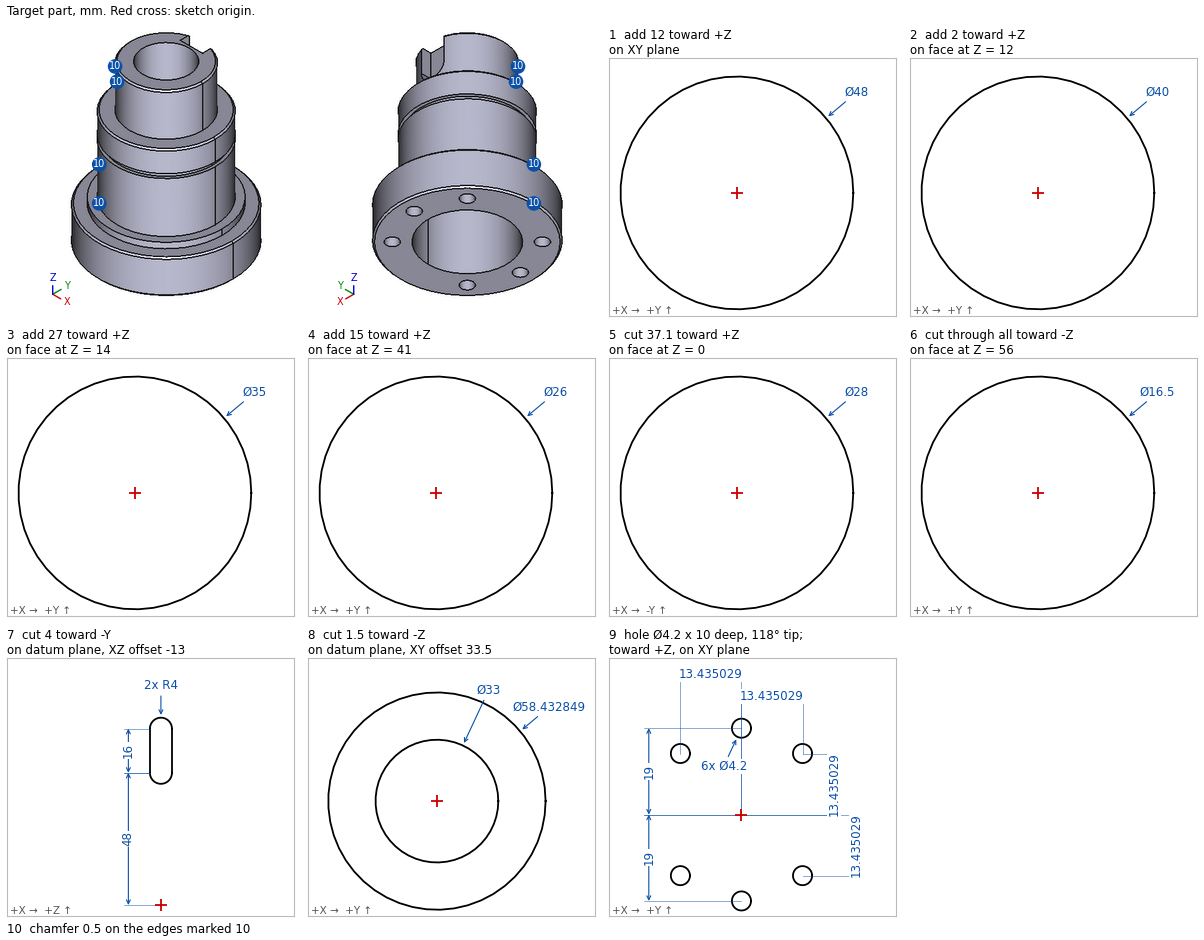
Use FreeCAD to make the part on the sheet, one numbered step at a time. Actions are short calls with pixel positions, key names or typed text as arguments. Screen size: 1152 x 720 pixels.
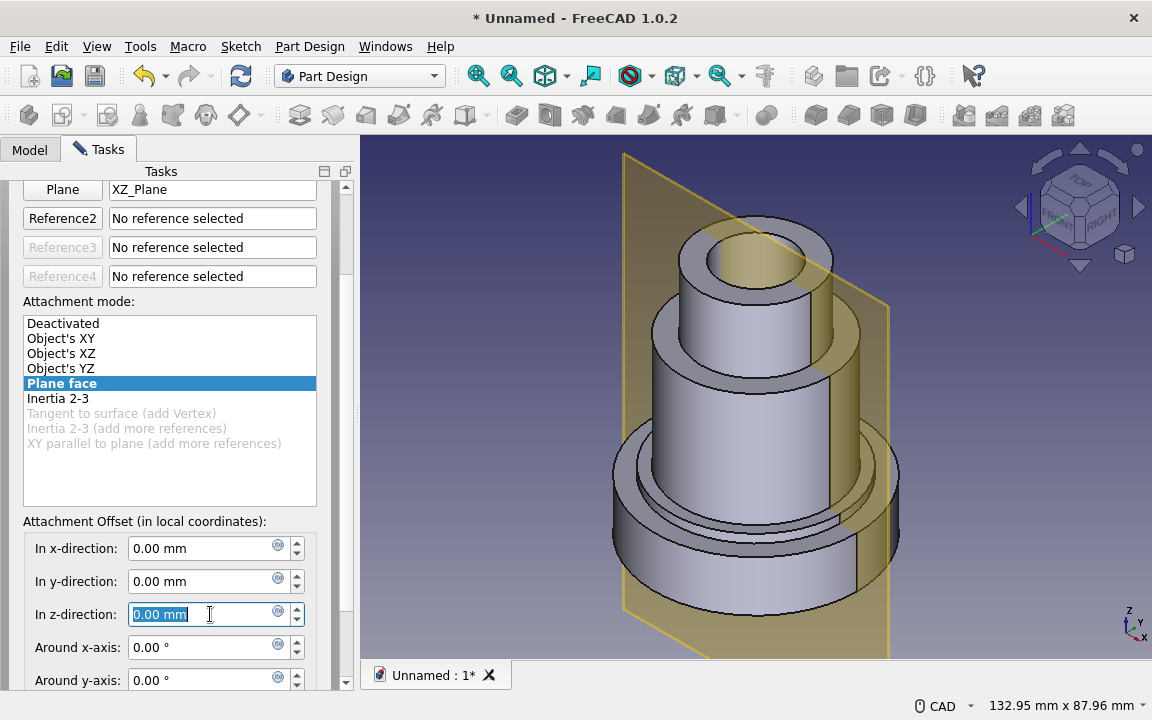
text(-13)
key(Tab)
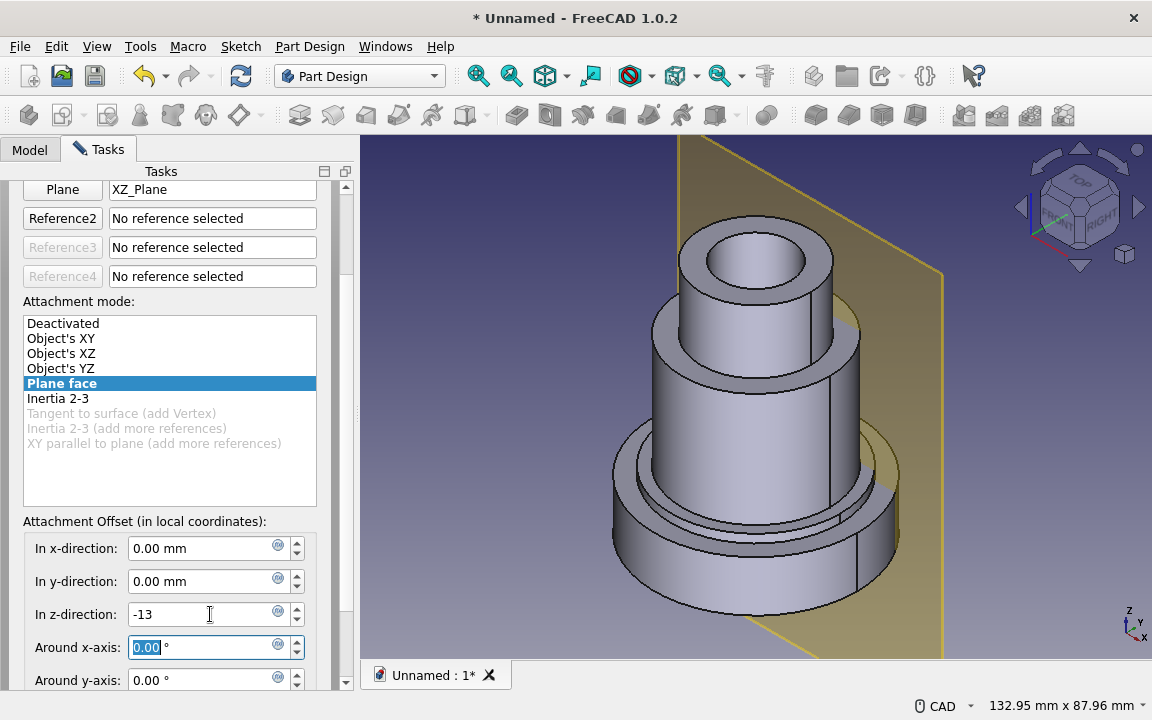
scroll(346, 436, up, 3)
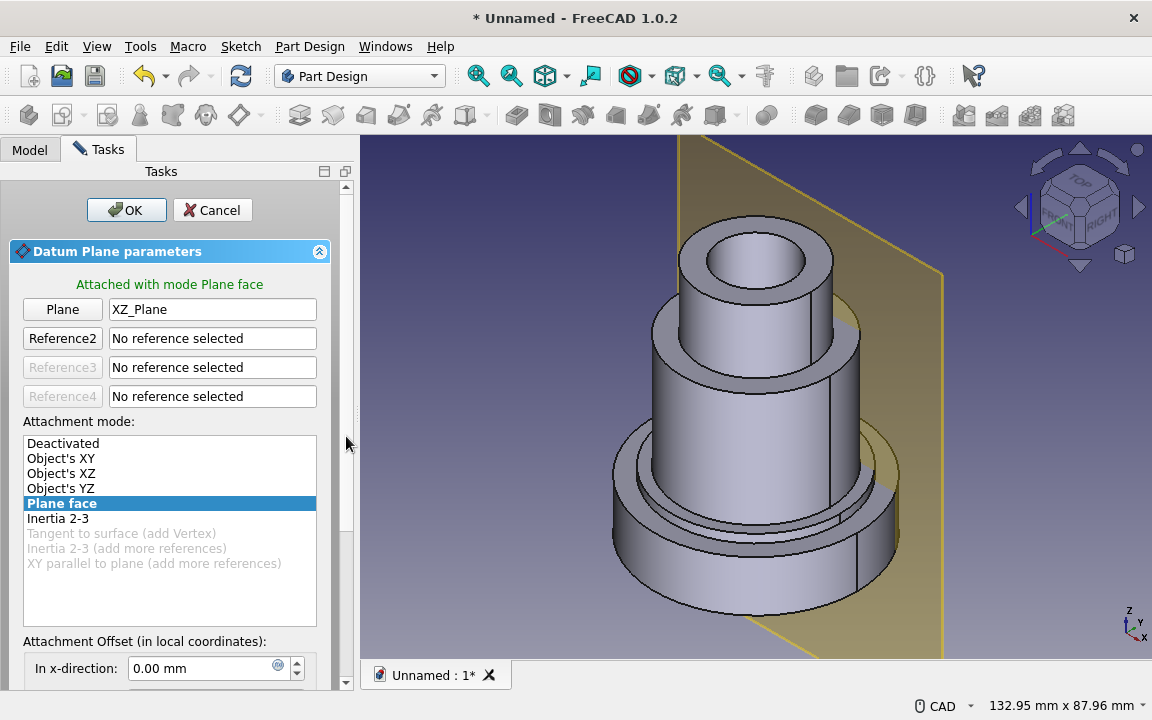
click(127, 210)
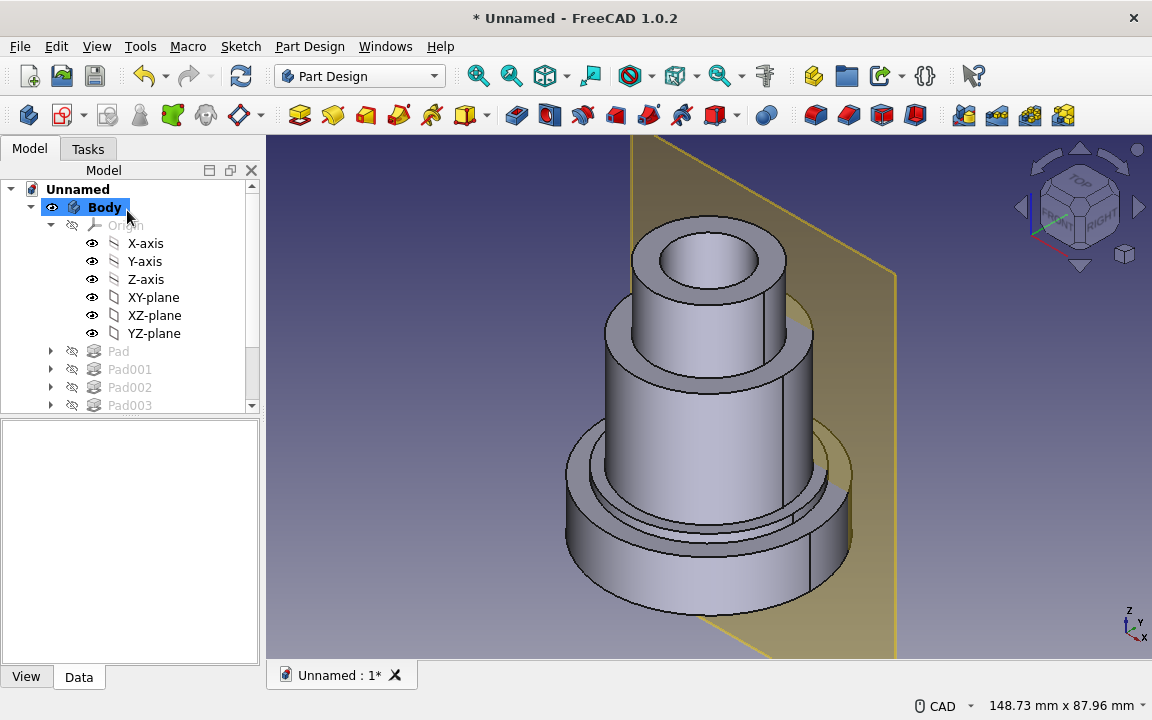
scroll(101, 293, down, 3)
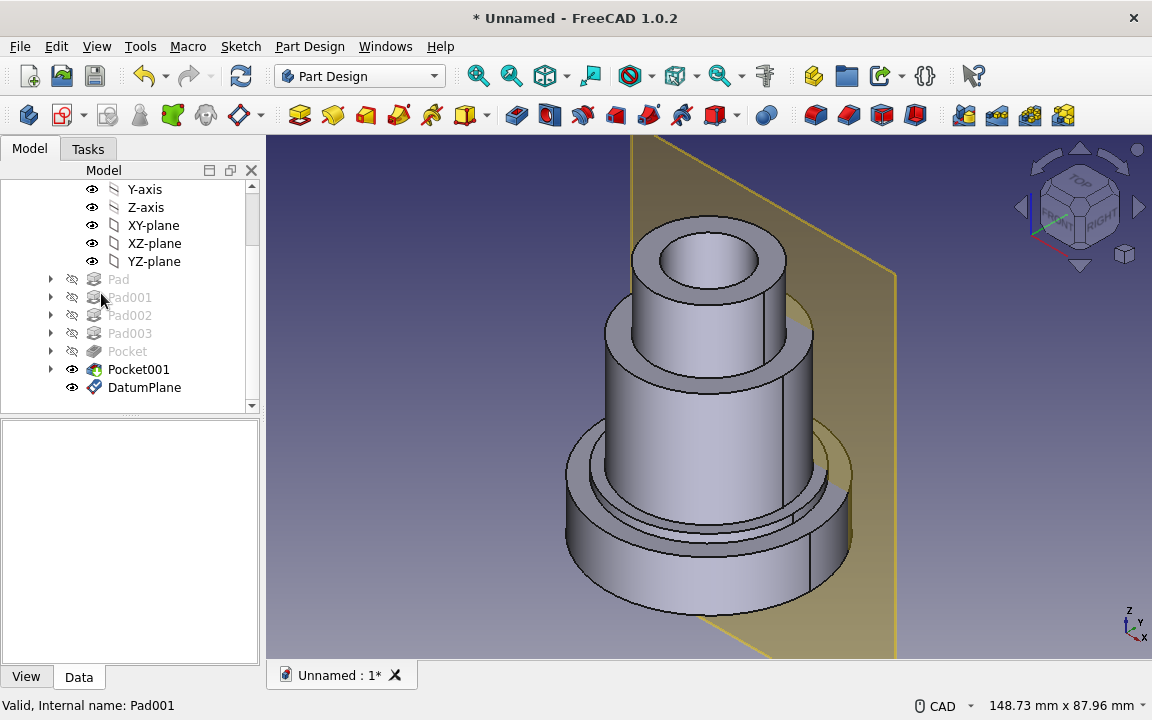
click(117, 387)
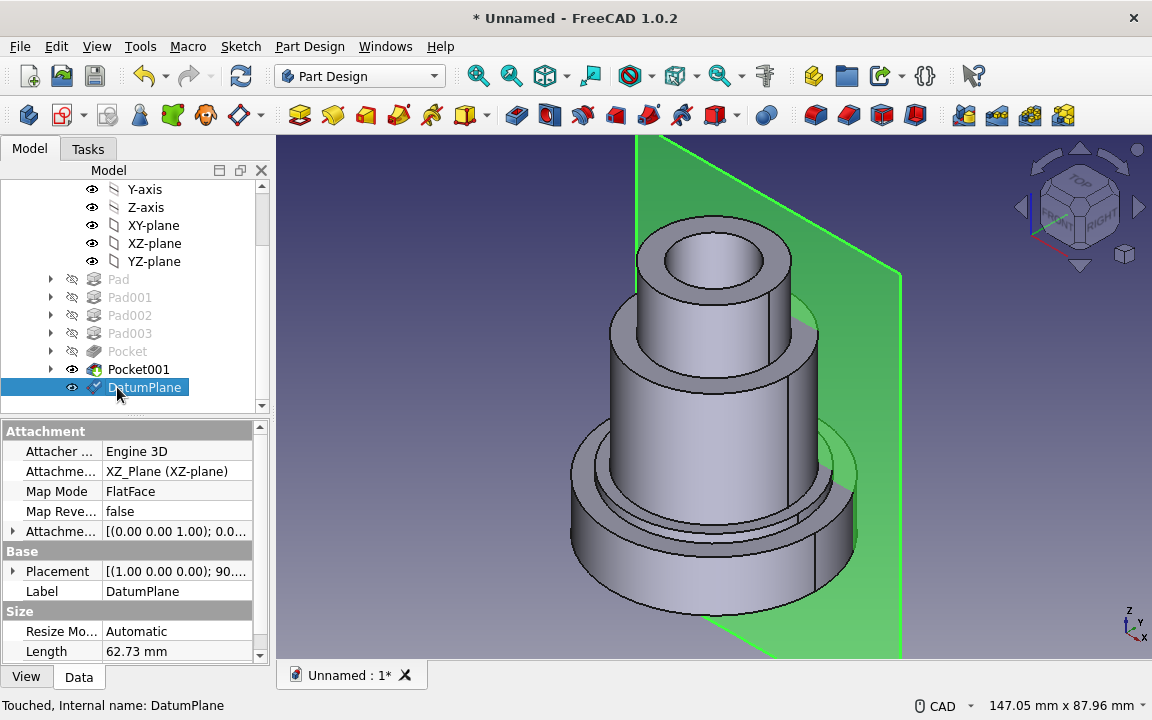
click(62, 116)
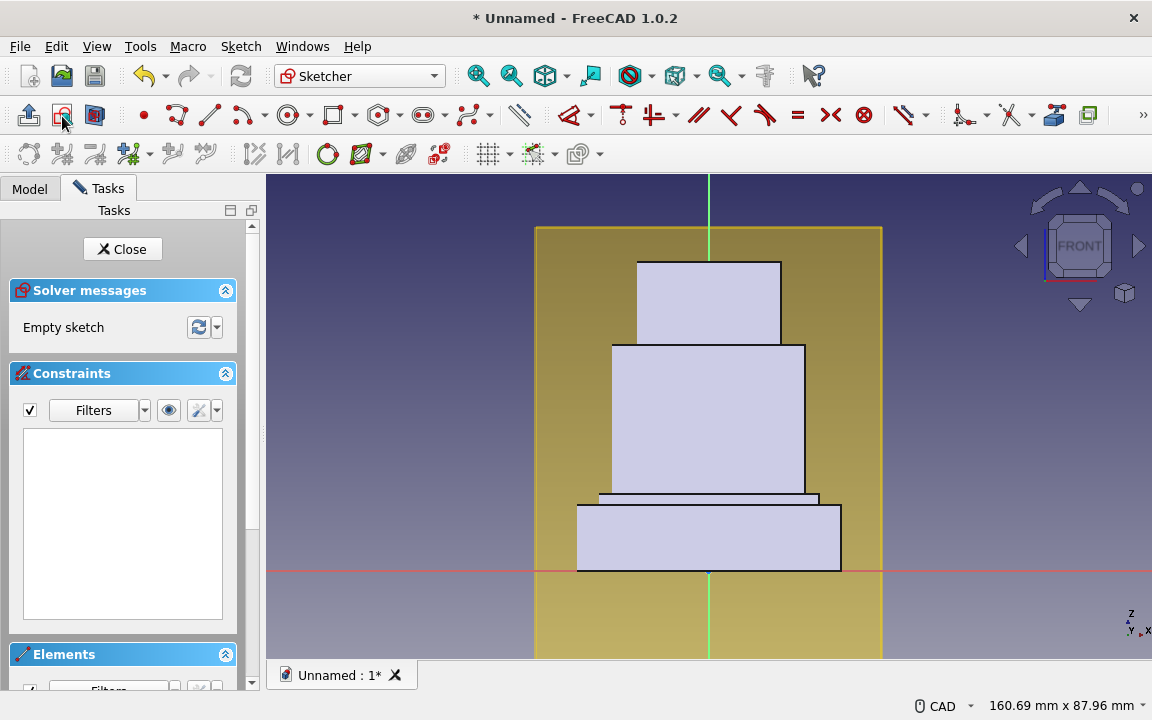
key(q)
key(s)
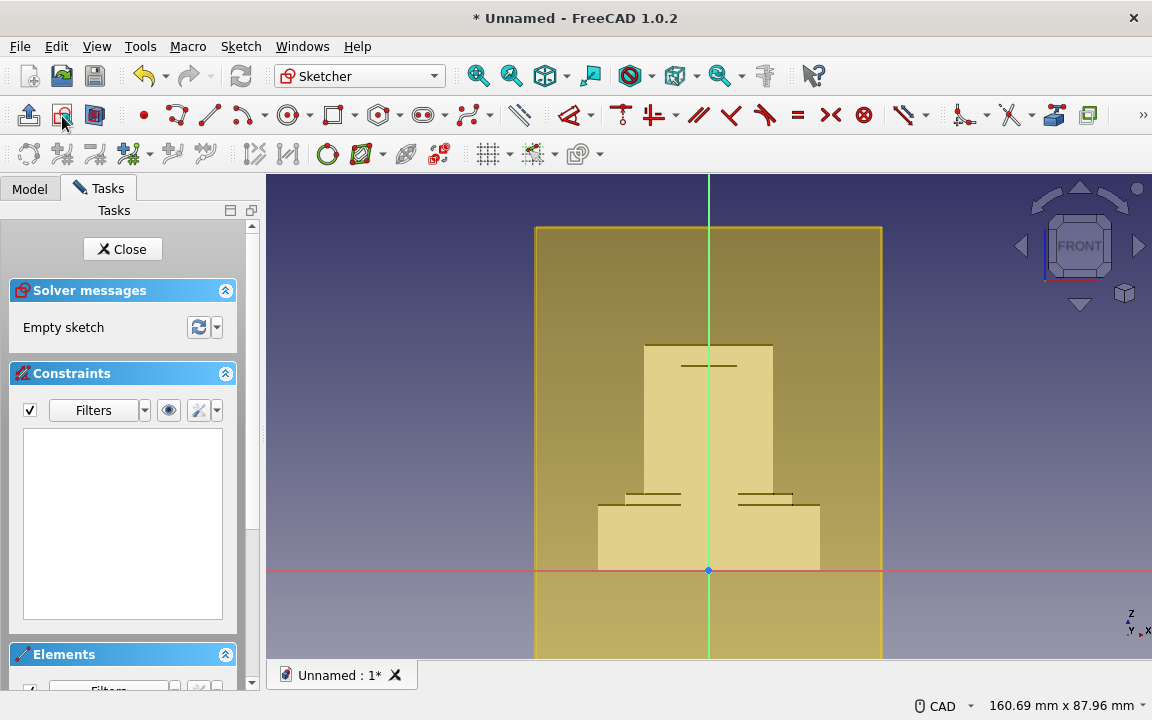
scroll(640, 416, down, 5)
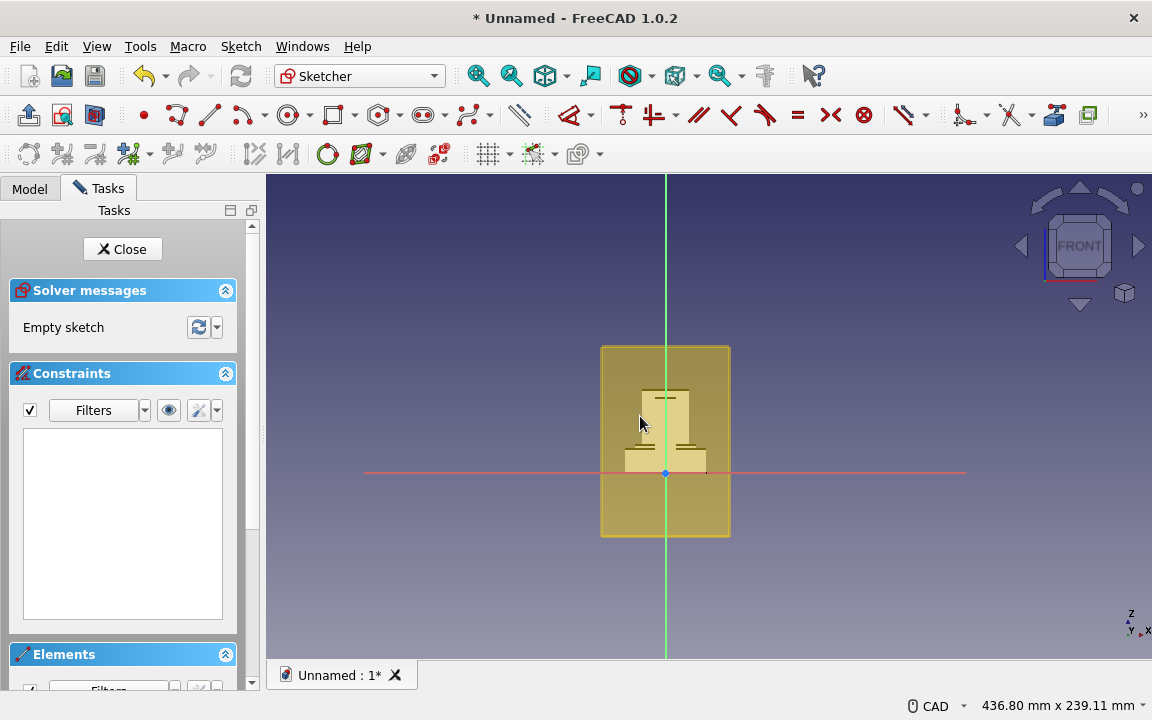
scroll(671, 348, up, 9)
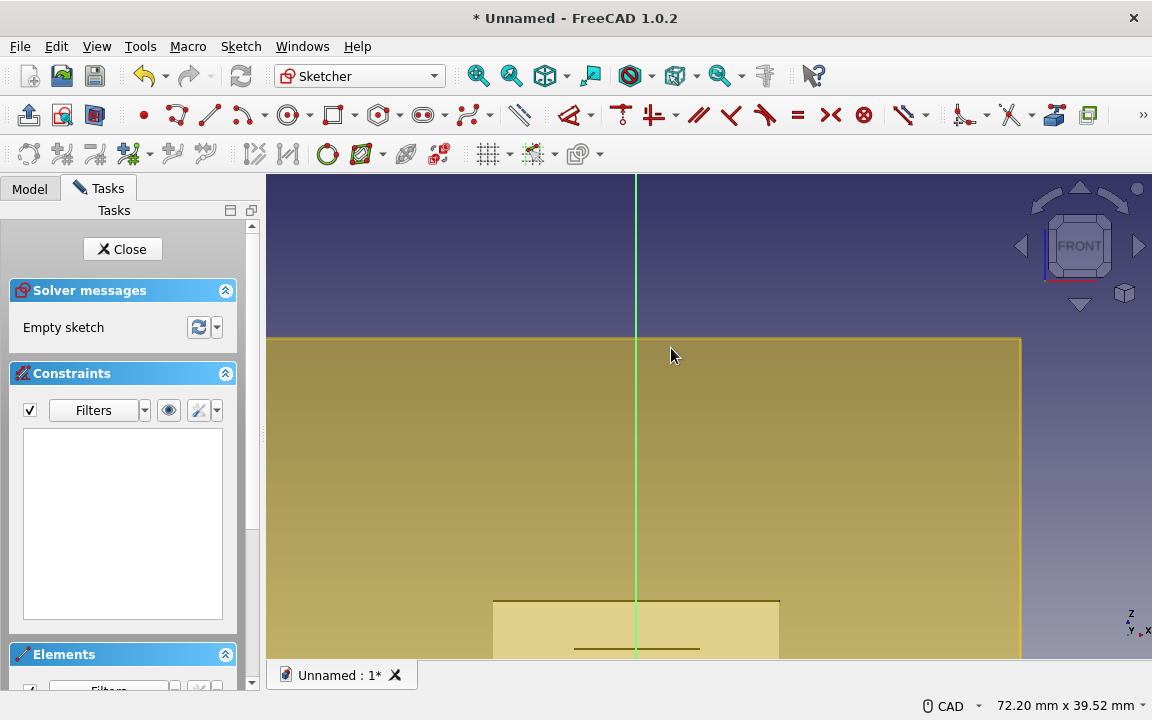
key(g)
key(s)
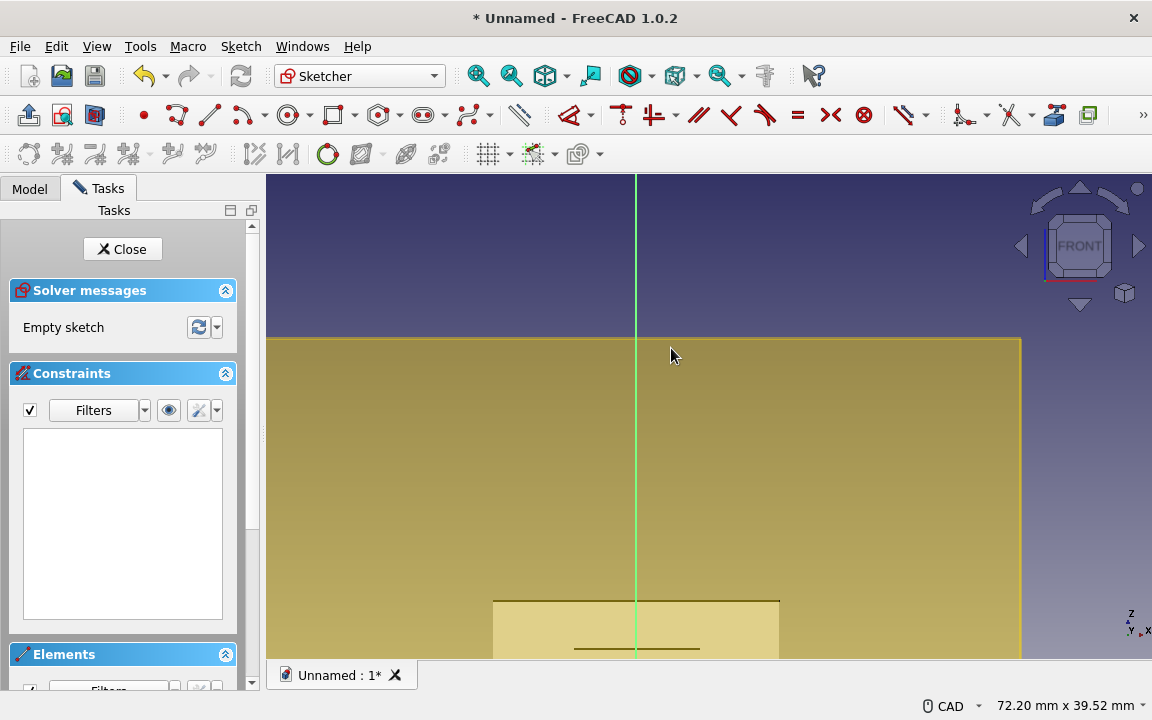
click(636, 515)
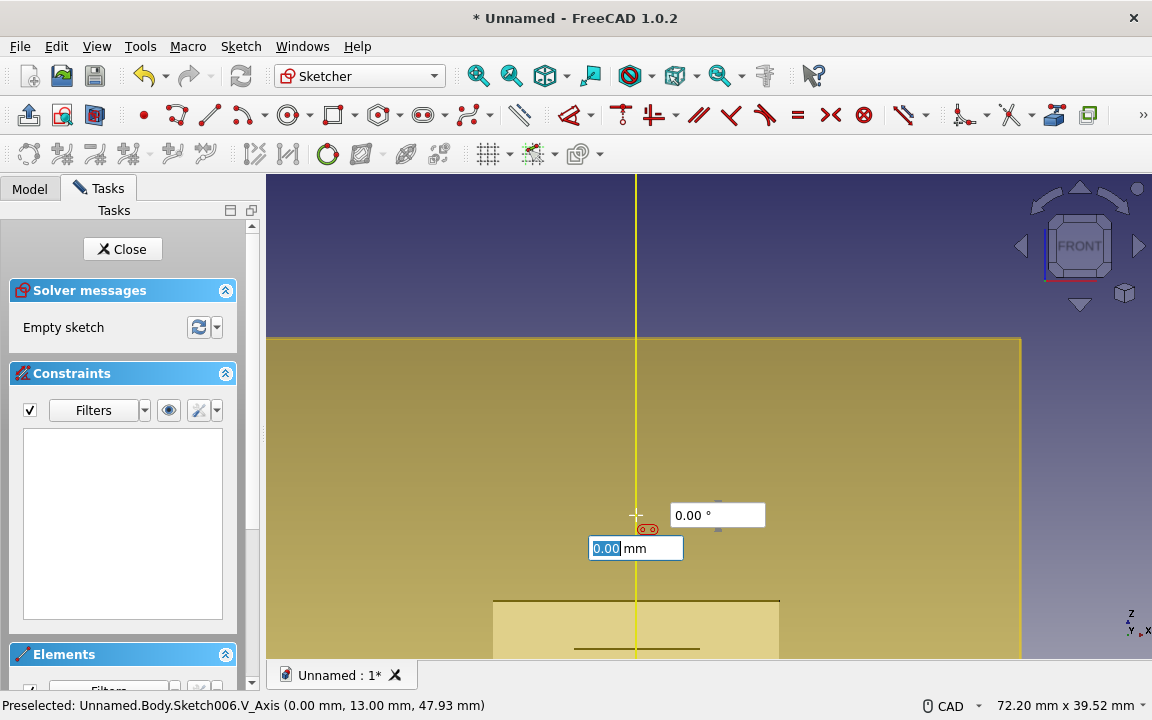
click(645, 319)